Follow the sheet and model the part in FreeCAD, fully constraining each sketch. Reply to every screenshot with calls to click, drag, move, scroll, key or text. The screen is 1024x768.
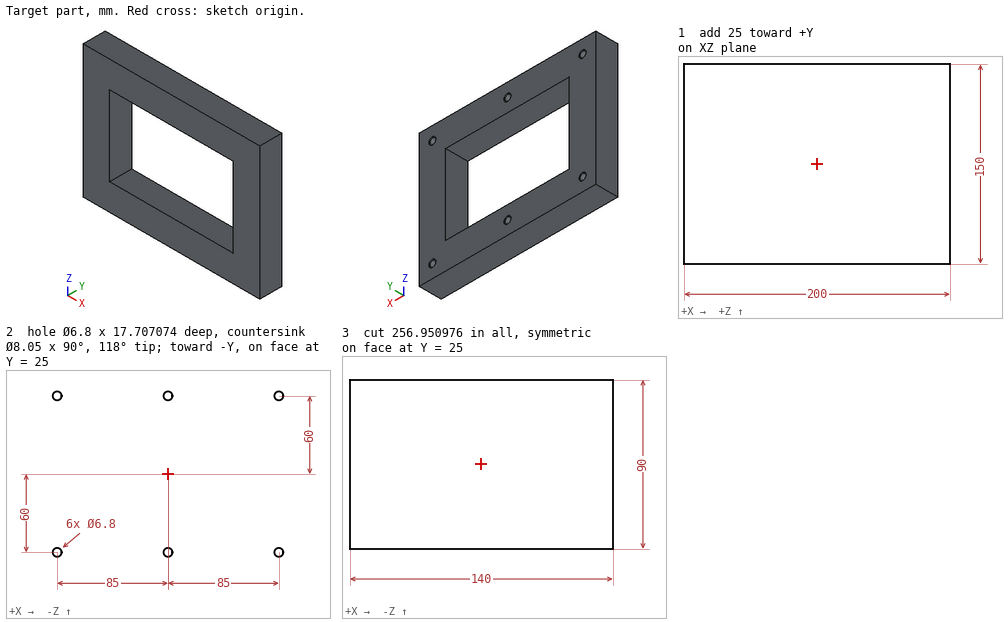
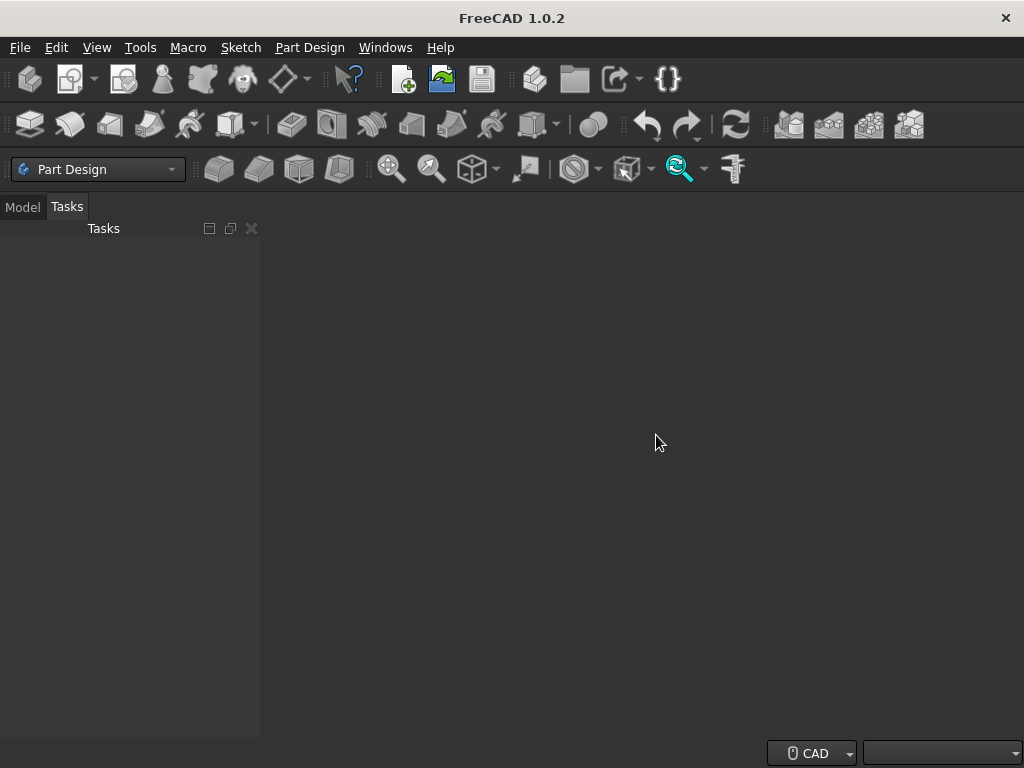
click(402, 80)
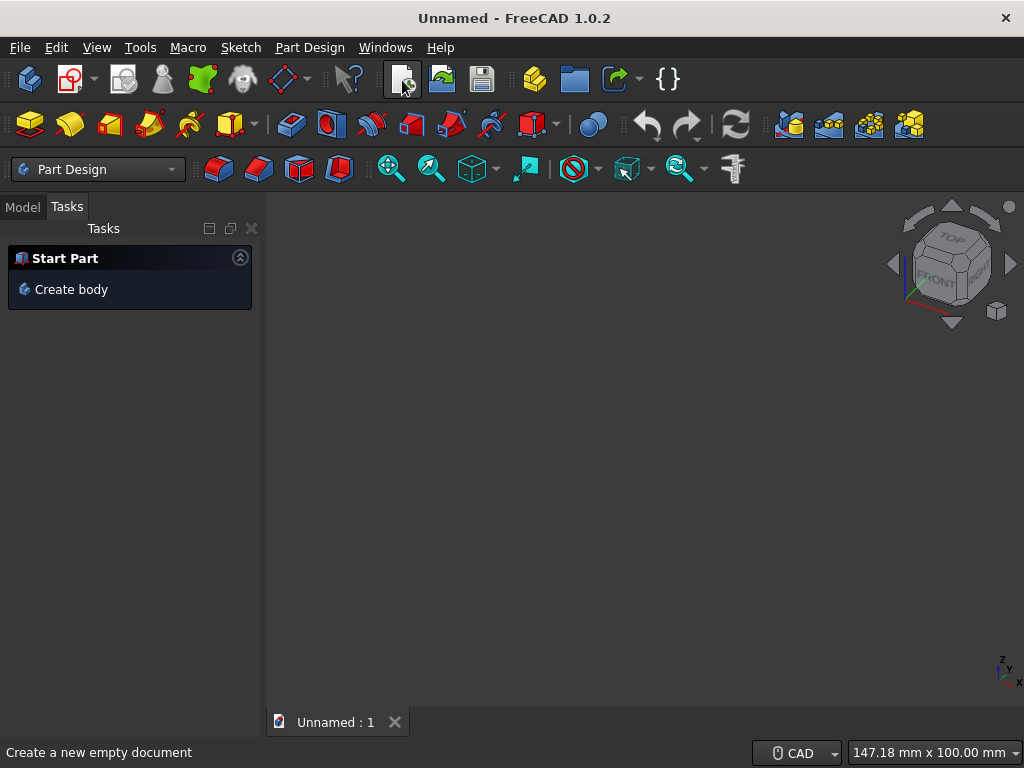
click(70, 80)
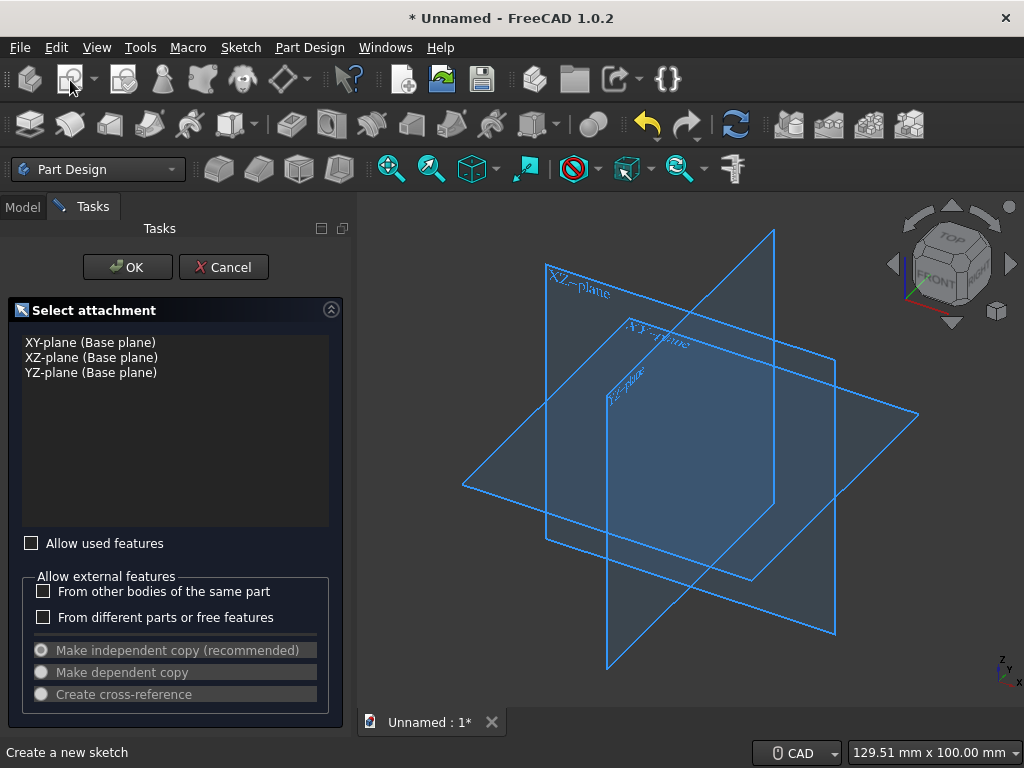
click(82, 358)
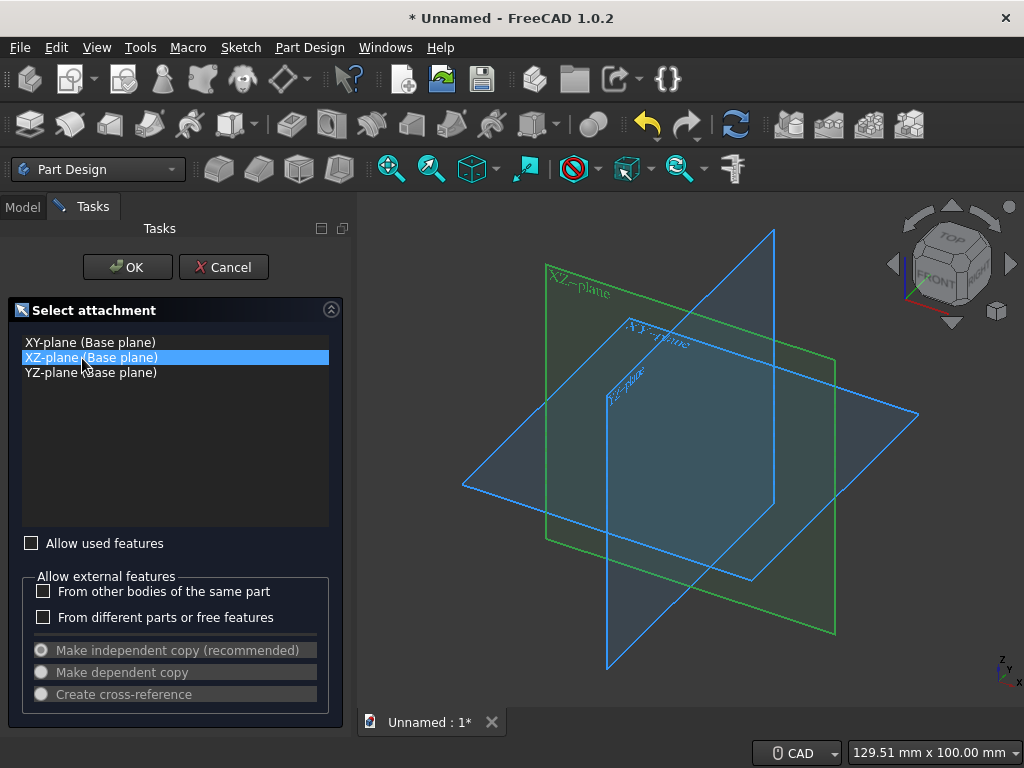
click(128, 267)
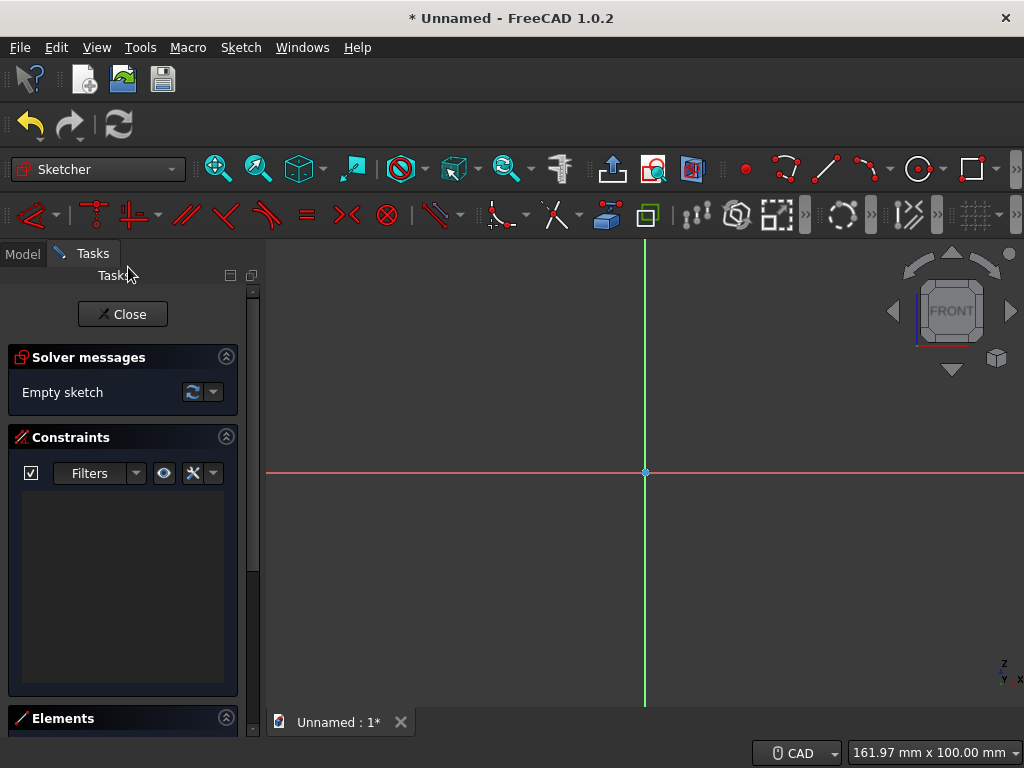
scroll(521, 473, down, 4)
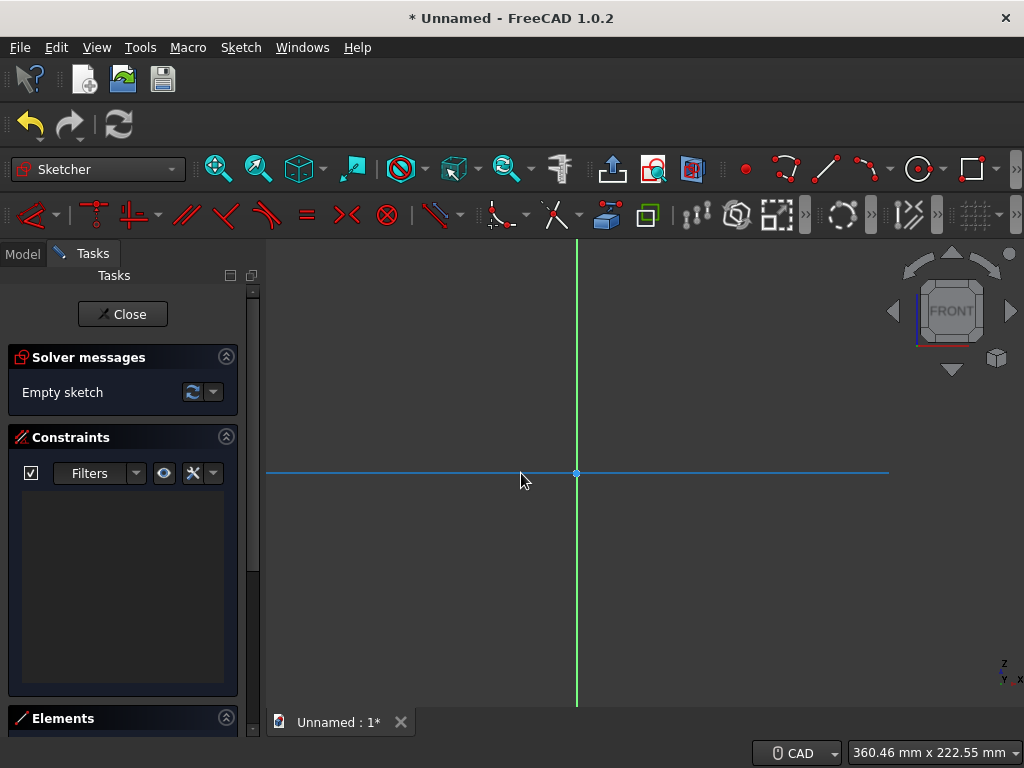
key(g)
key(v)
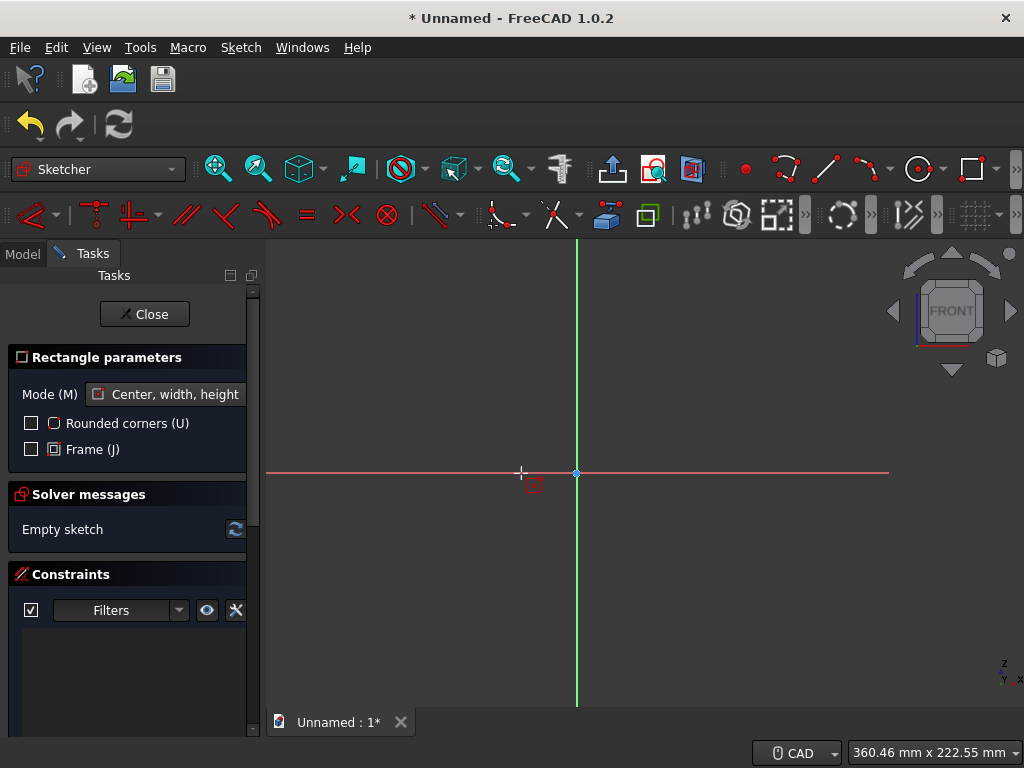
click(577, 473)
click(787, 316)
key(Escape)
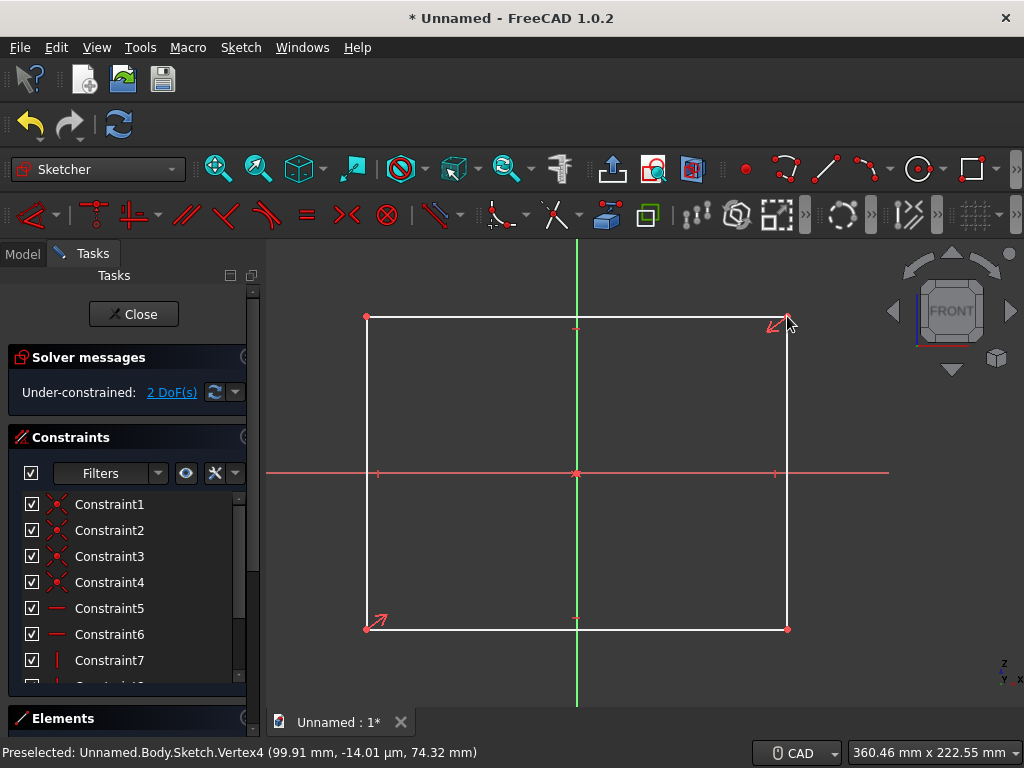
click(493, 630)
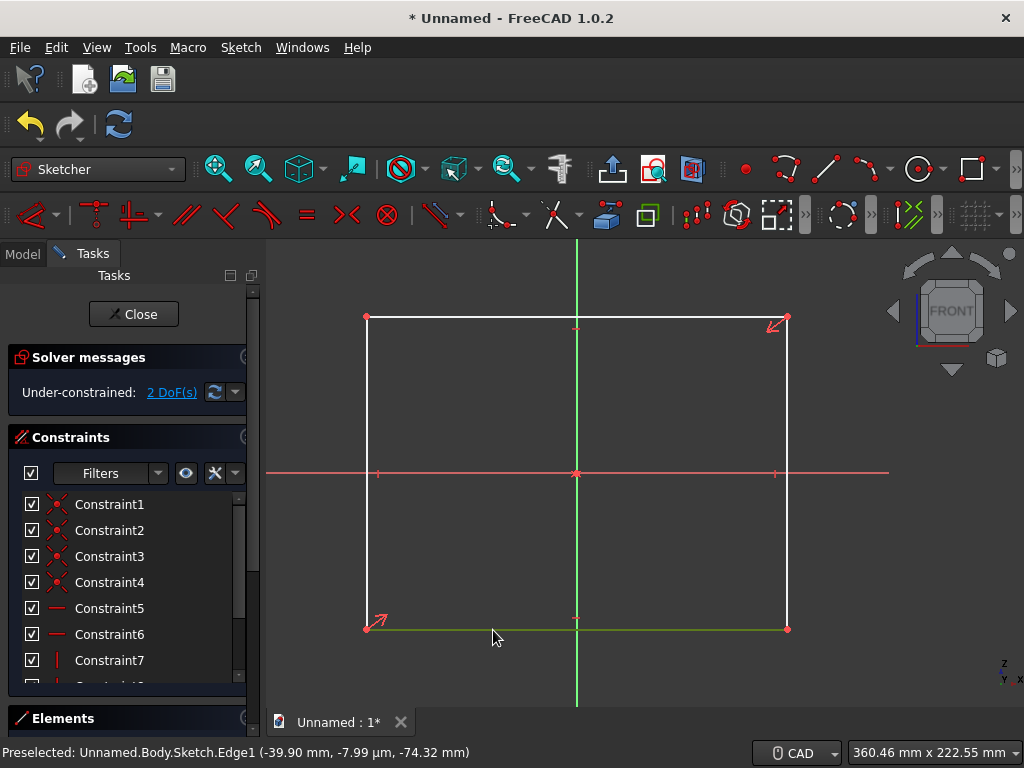
click(58, 216)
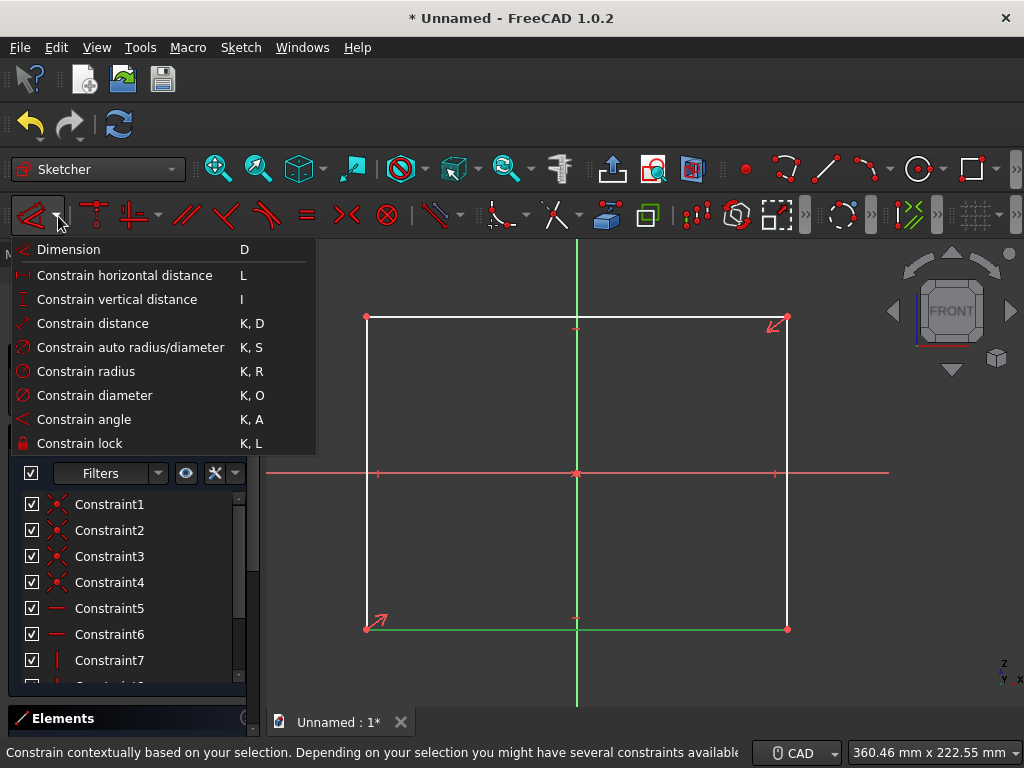
click(164, 275)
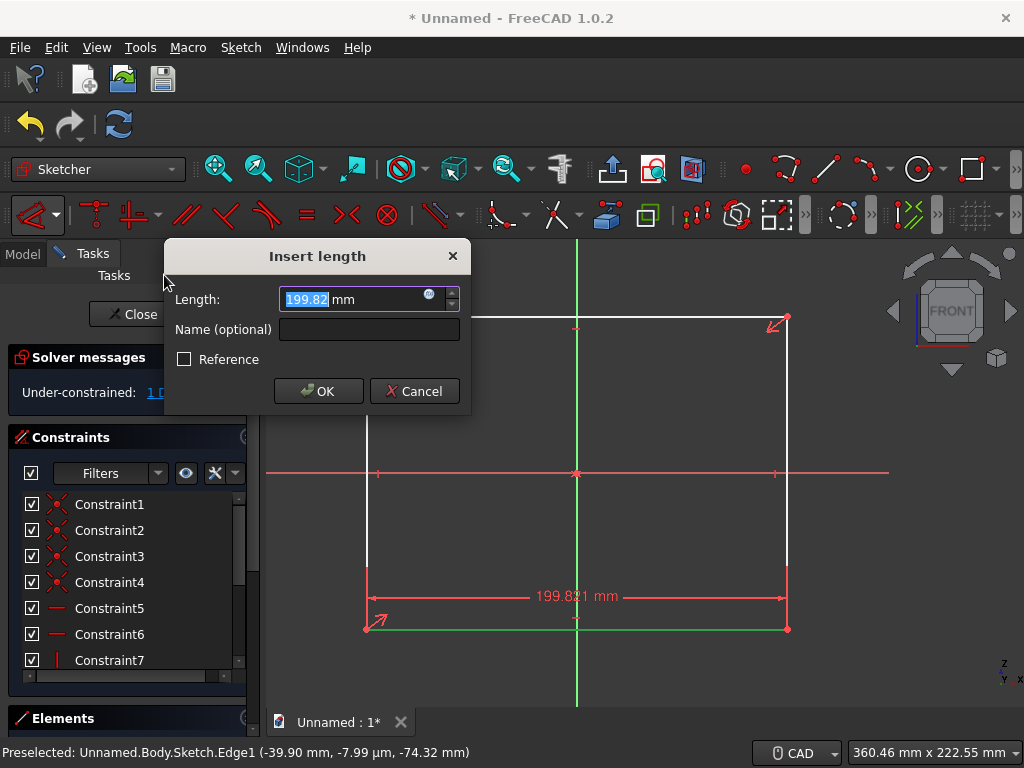
text(200)
key(Return)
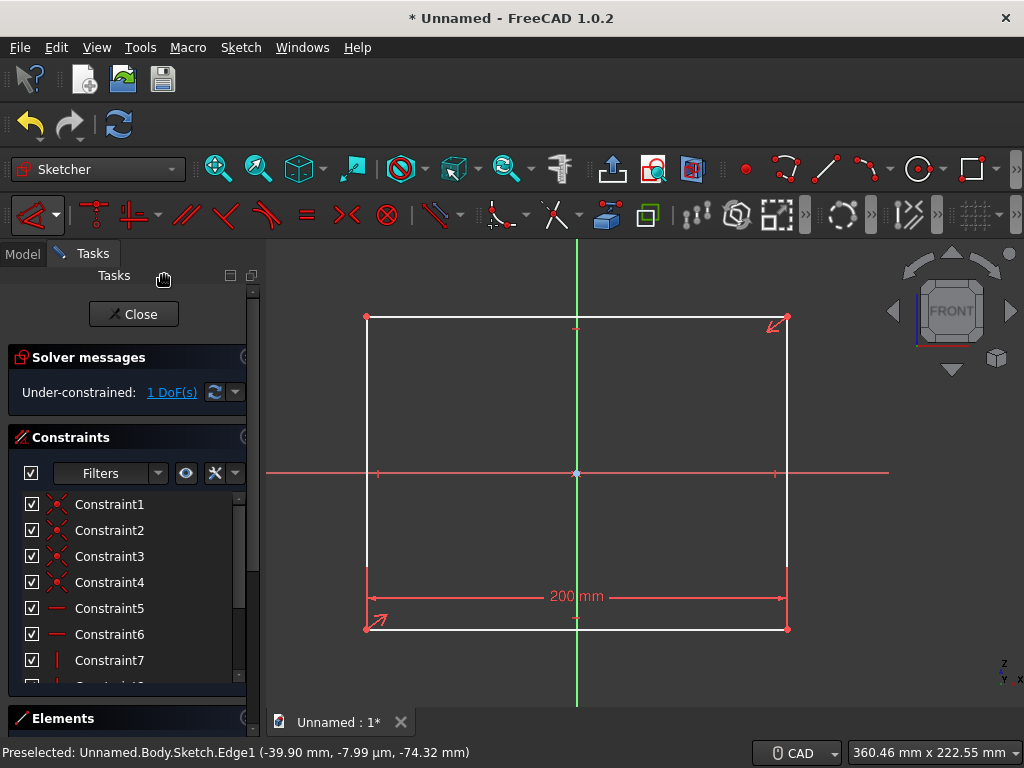
click(787, 536)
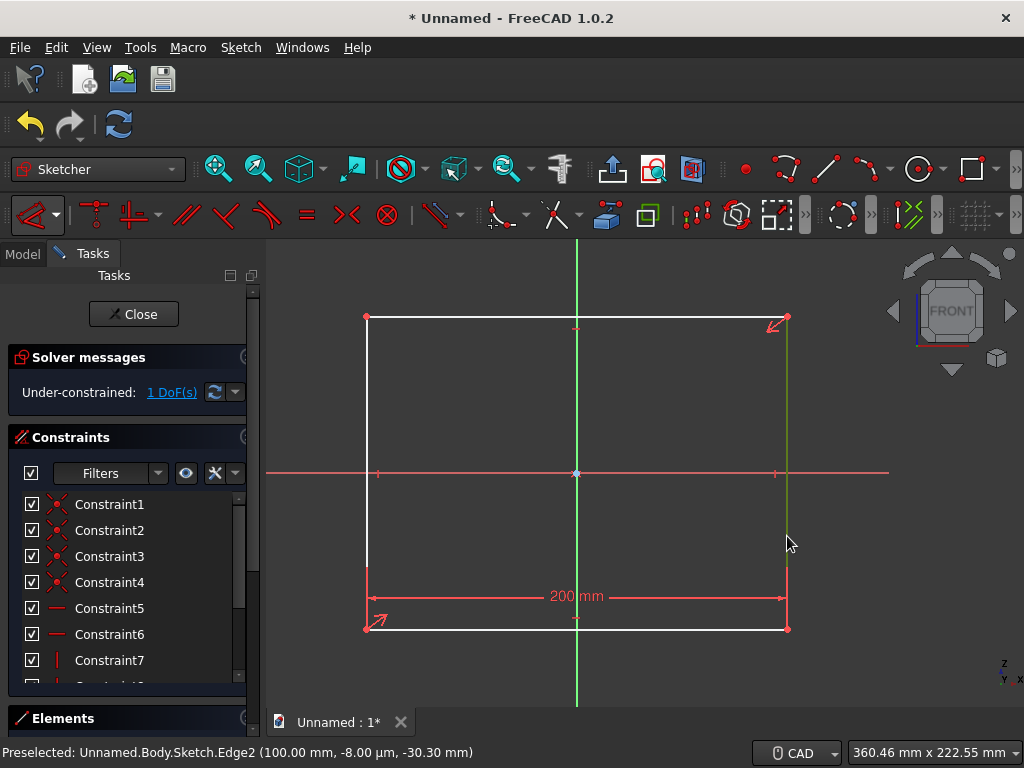
key(i)